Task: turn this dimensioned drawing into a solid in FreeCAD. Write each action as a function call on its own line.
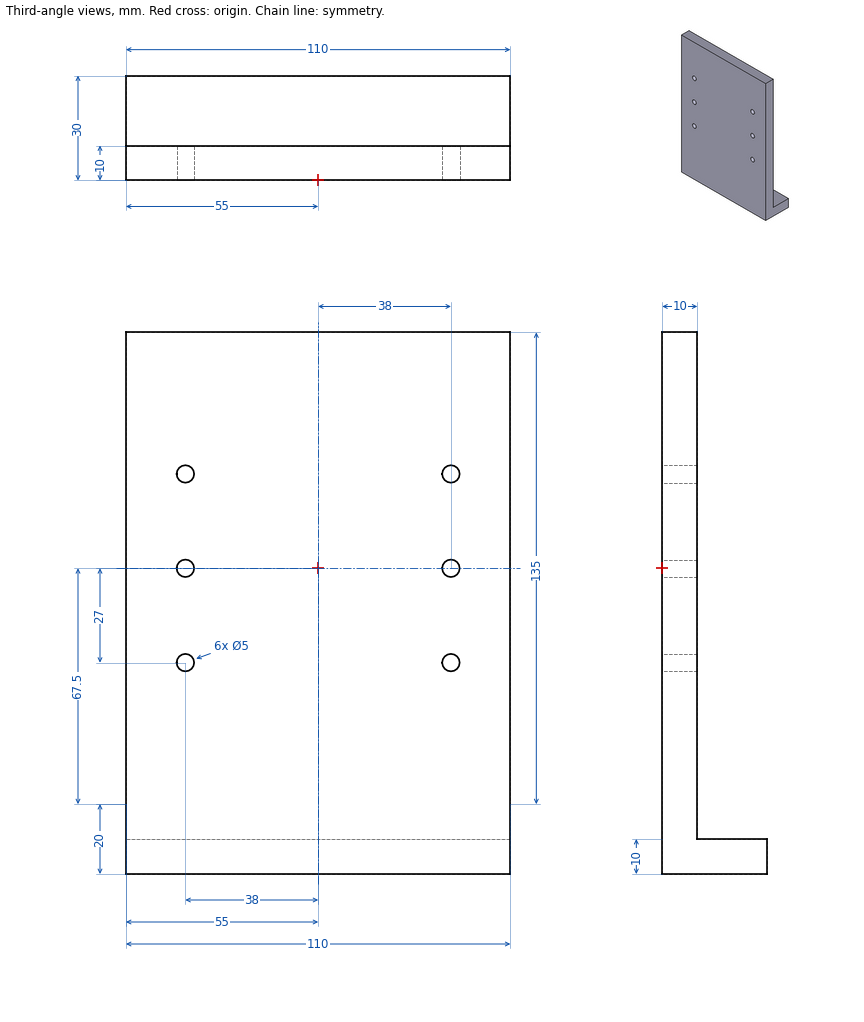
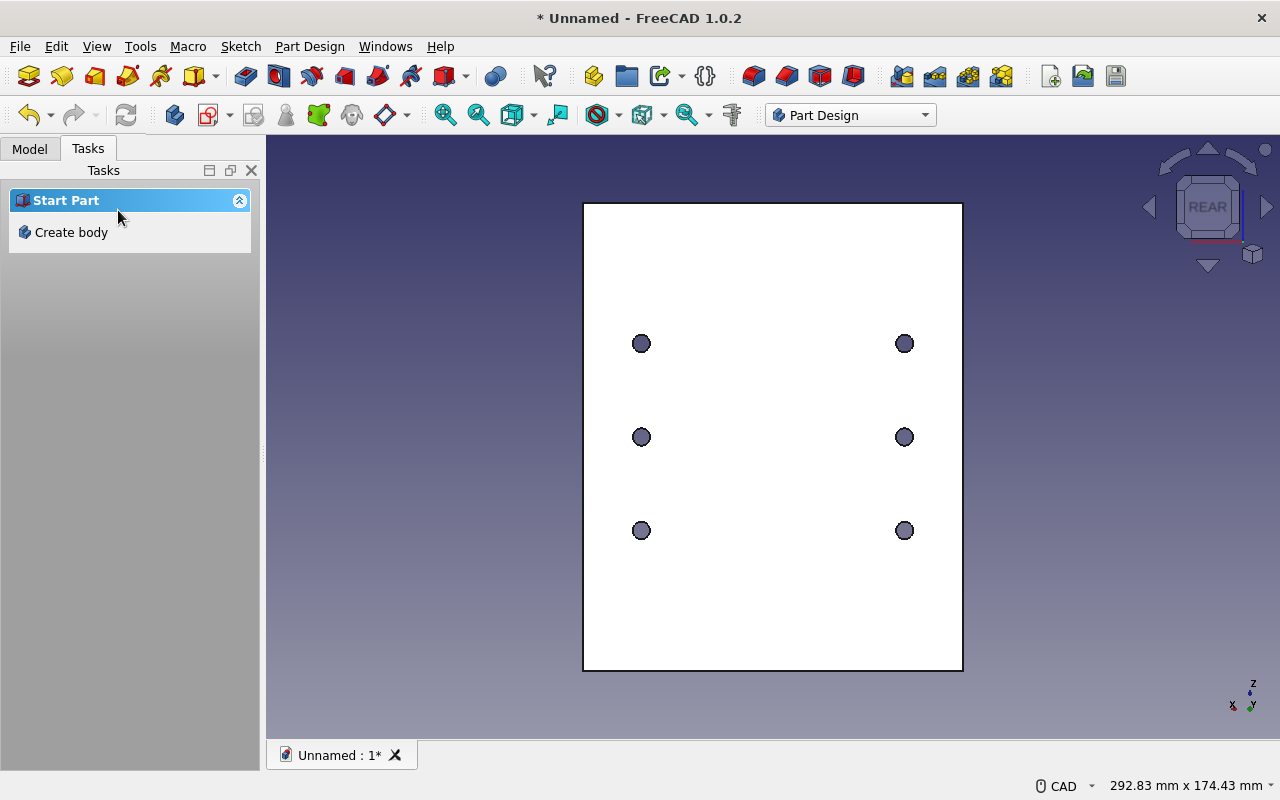
key(0)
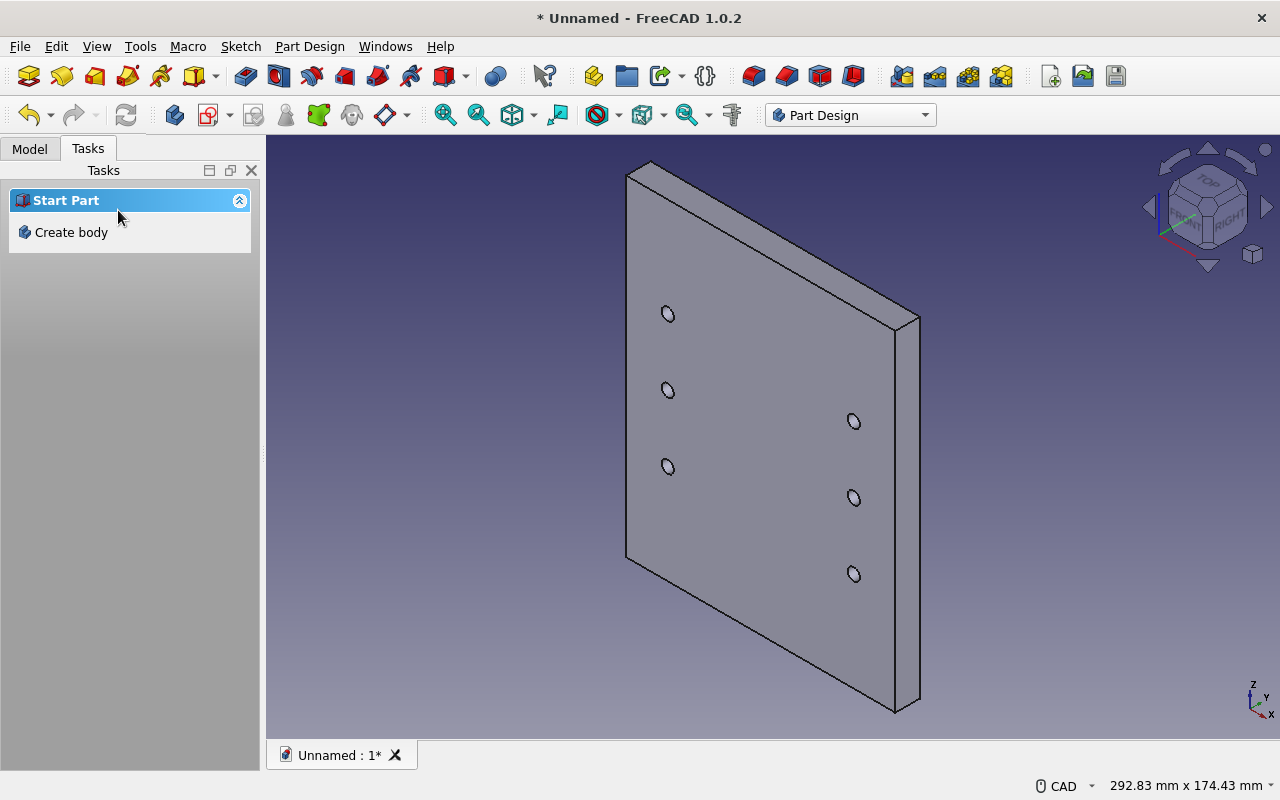
click(761, 498)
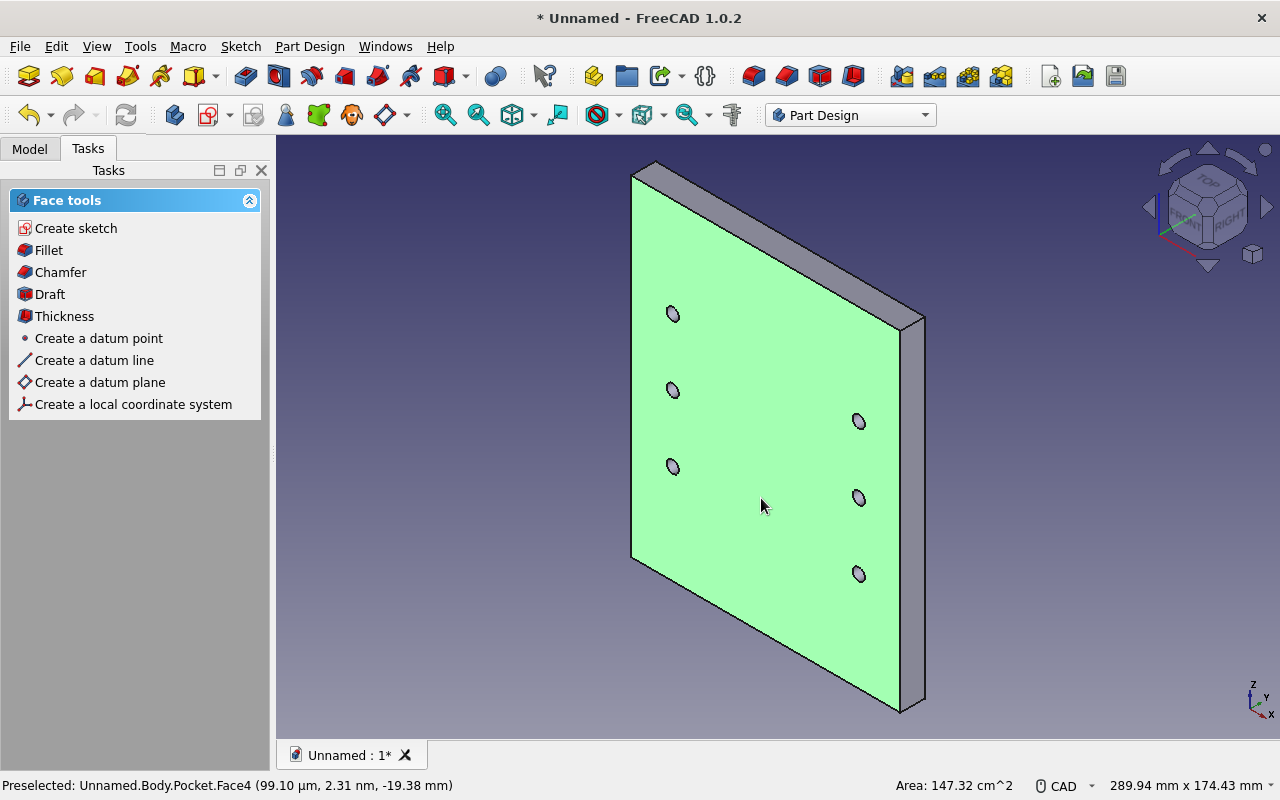
click(208, 116)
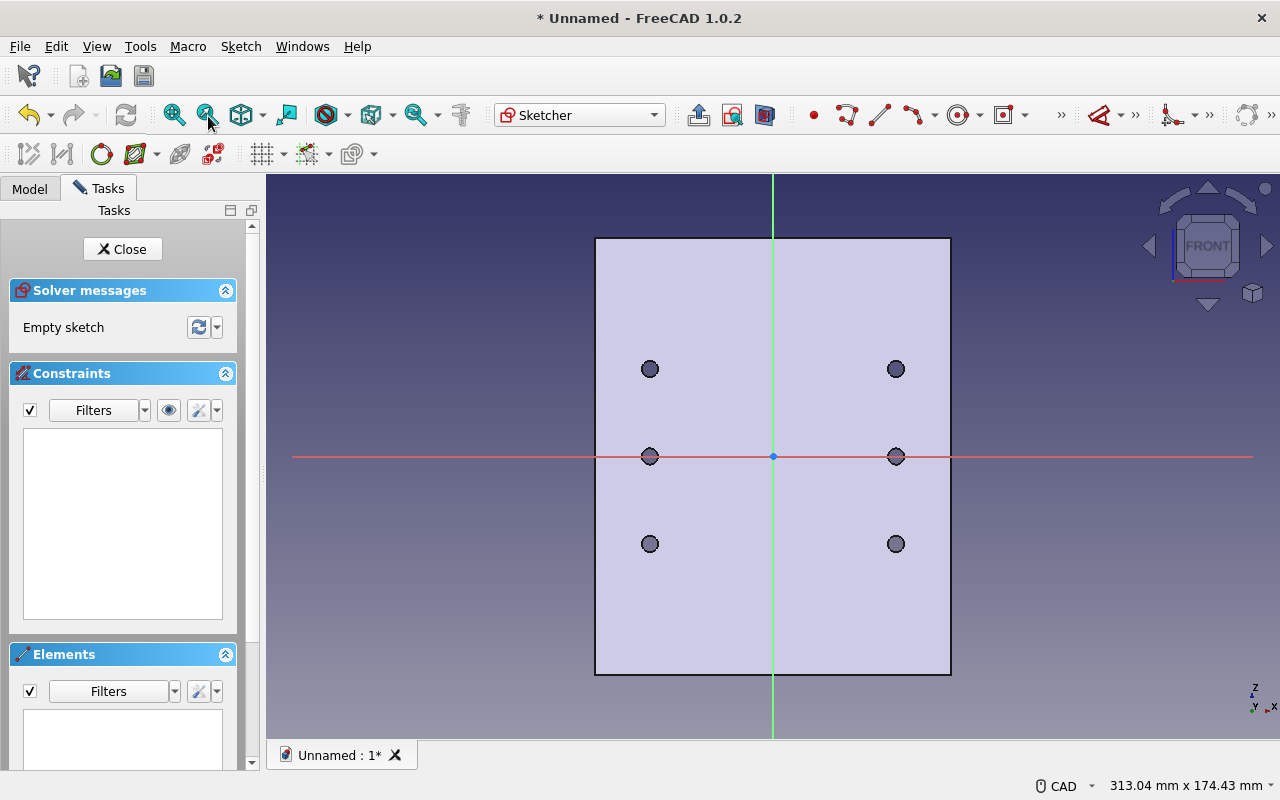
scroll(395, 202, down, 1)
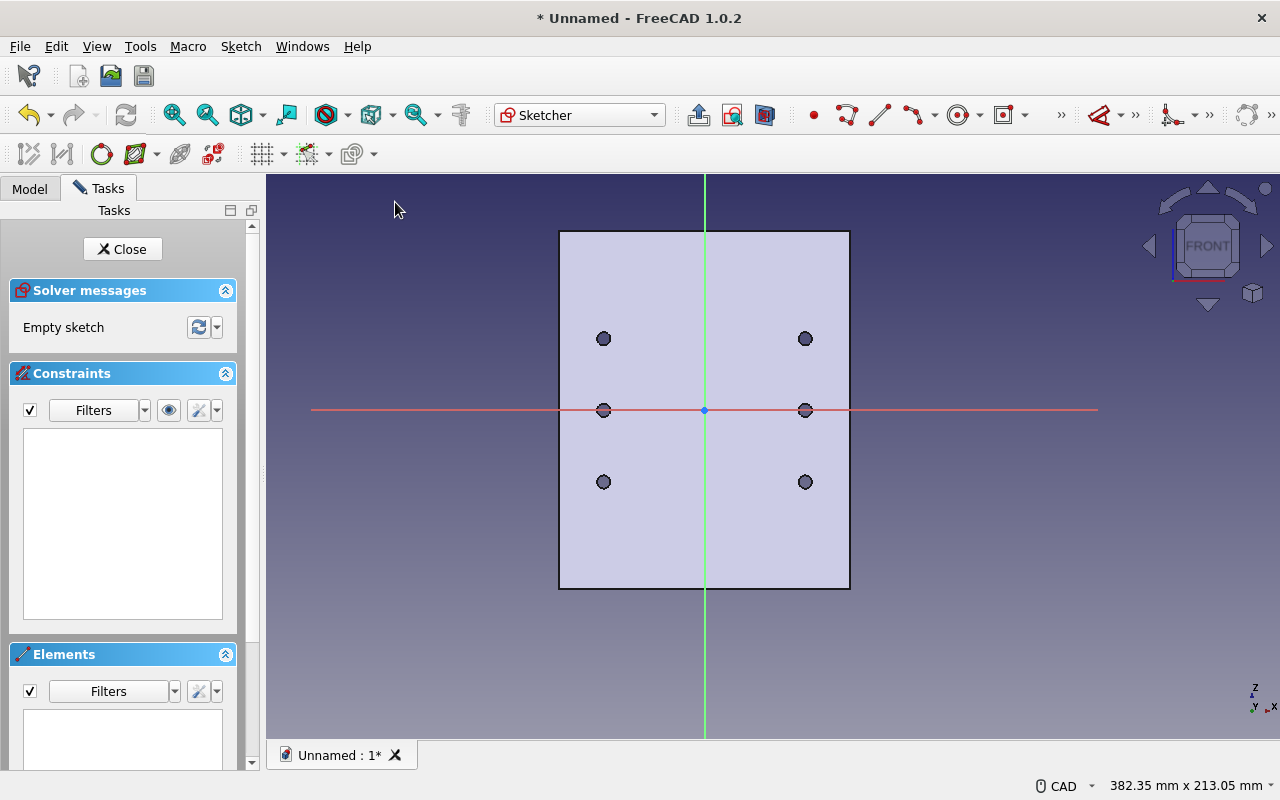
scroll(705, 669, up, 2)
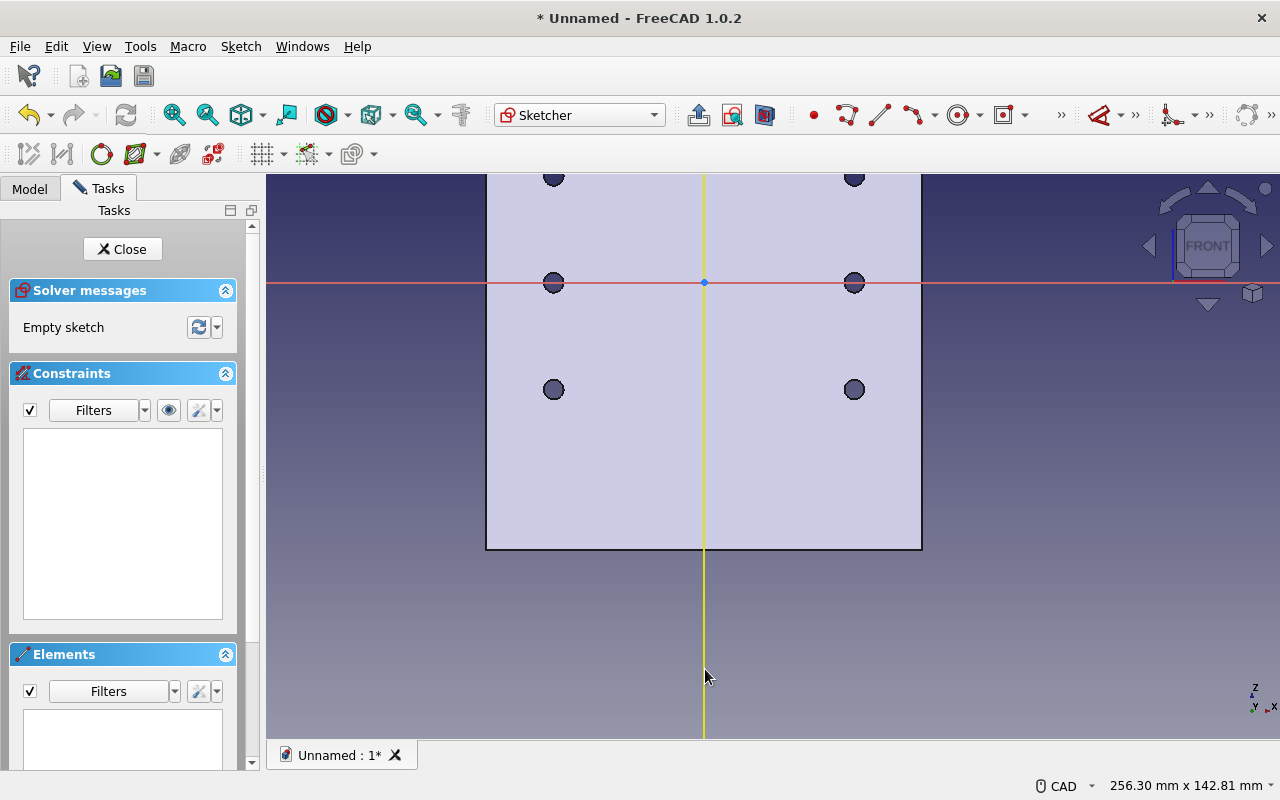
key(g)
key(r)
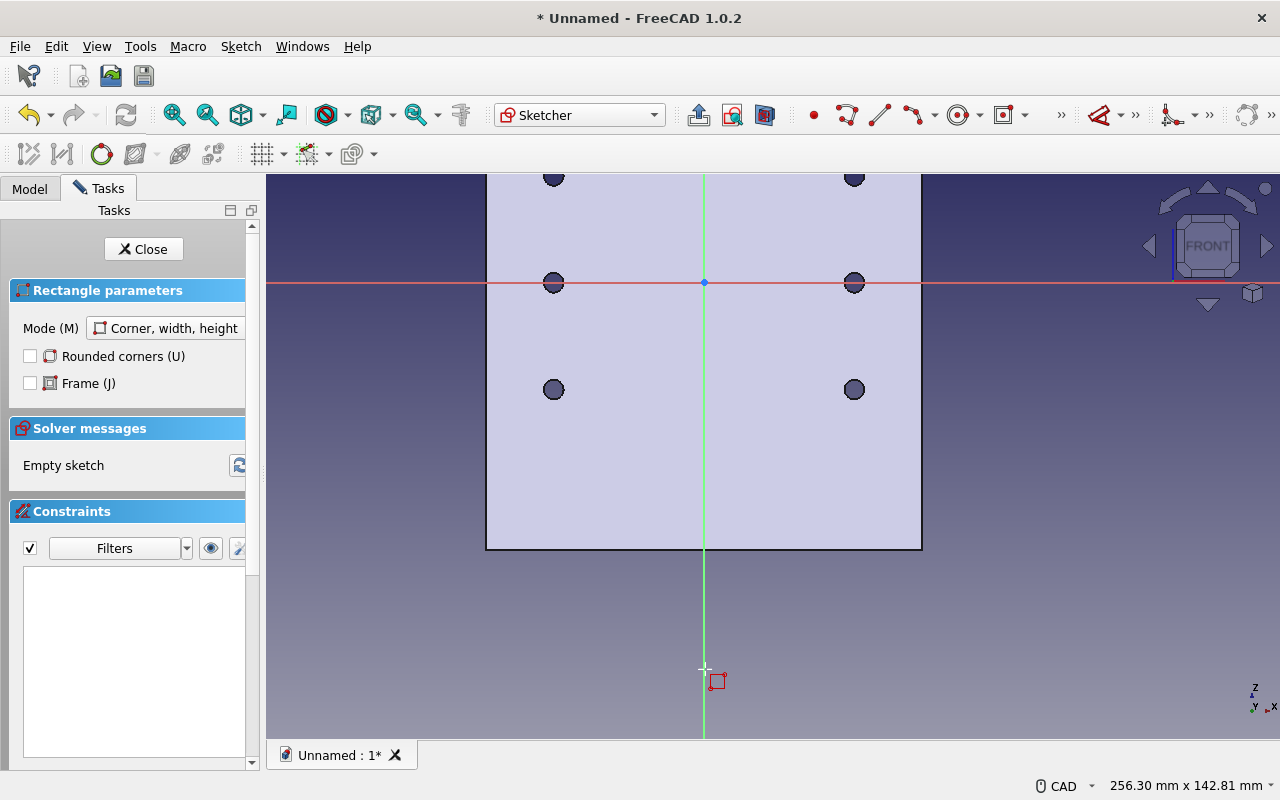
click(486, 550)
click(922, 629)
key(Escape)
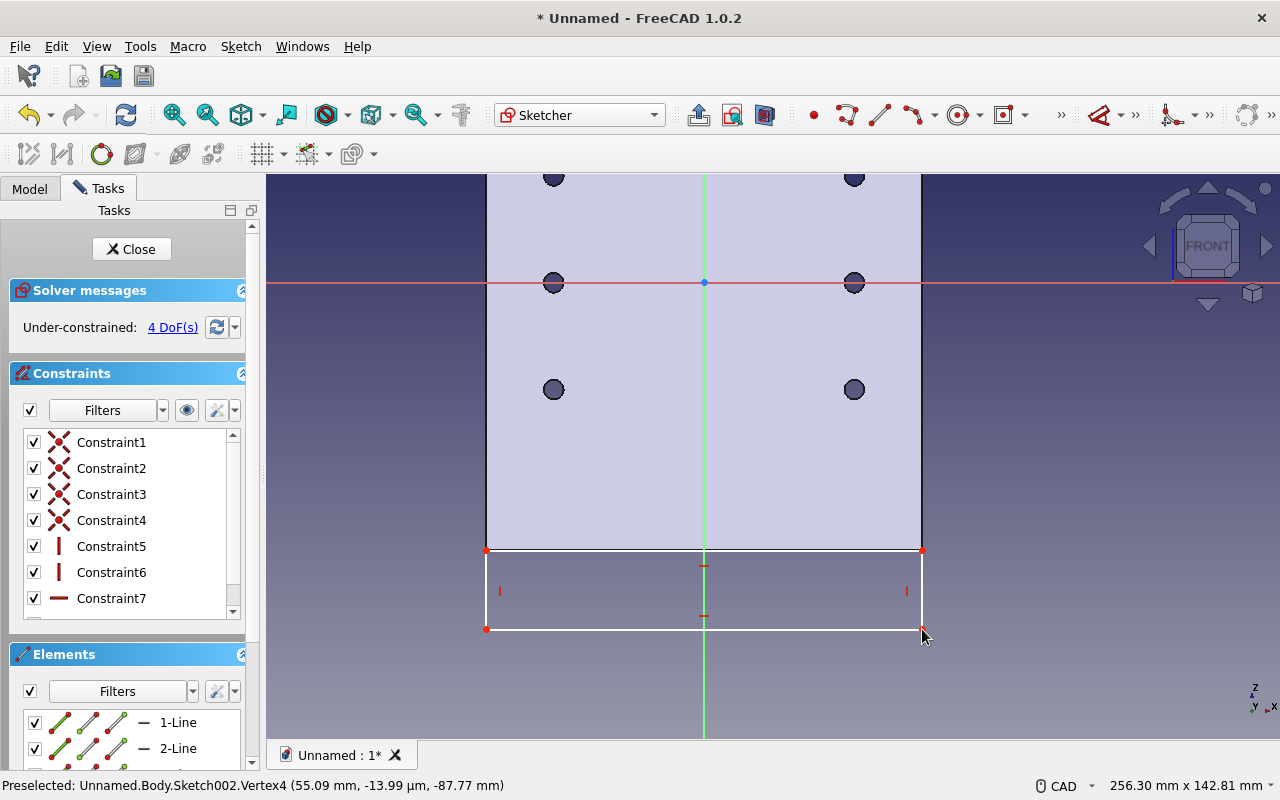
click(1098, 116)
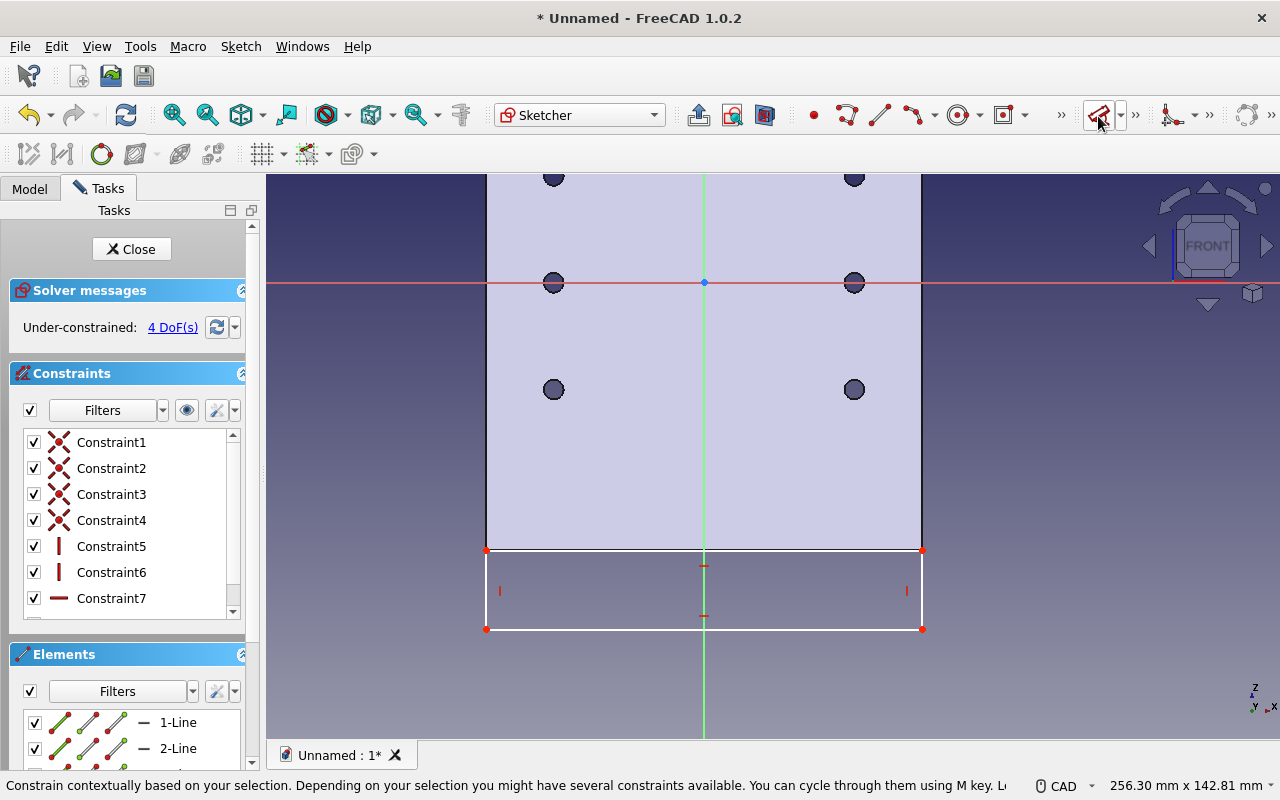
click(486, 575)
click(452, 590)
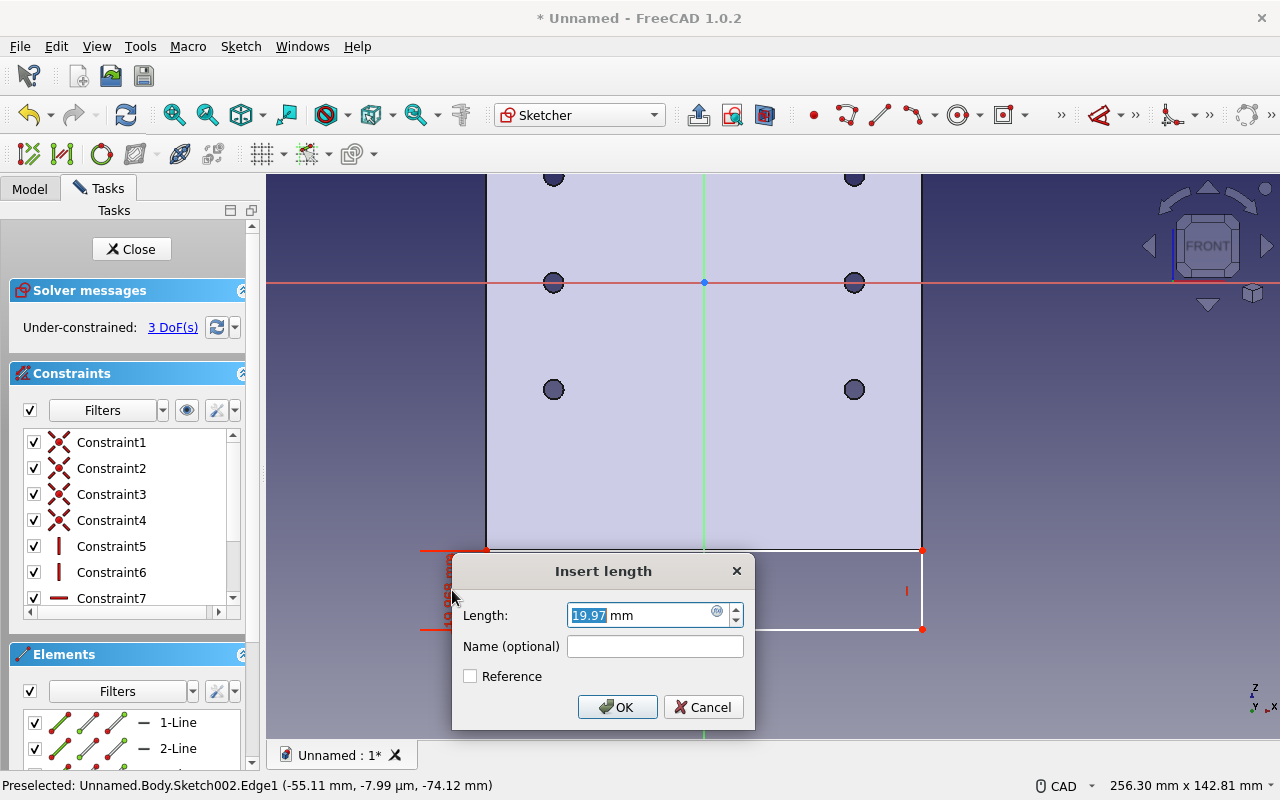
text(20)
key(Return)